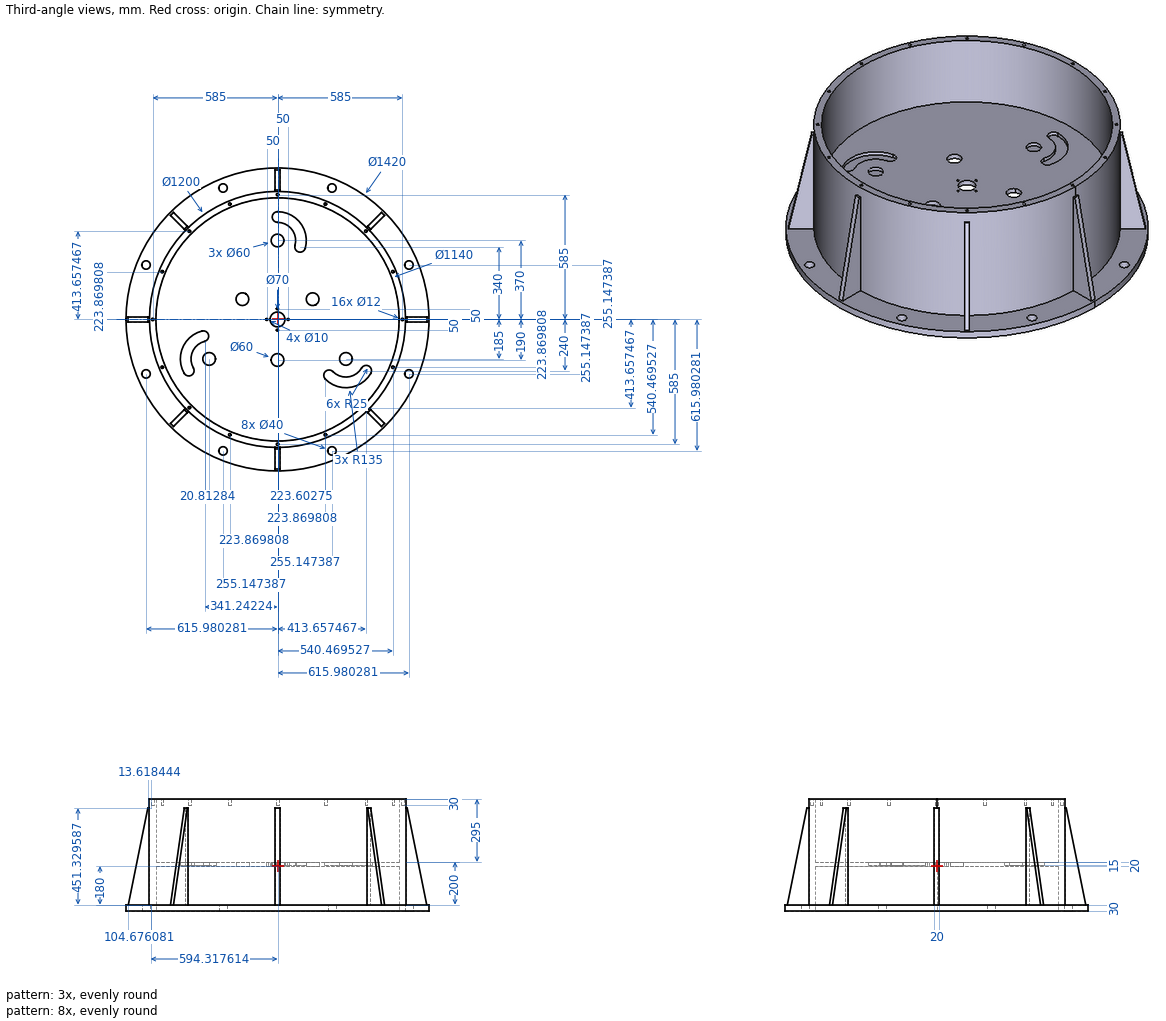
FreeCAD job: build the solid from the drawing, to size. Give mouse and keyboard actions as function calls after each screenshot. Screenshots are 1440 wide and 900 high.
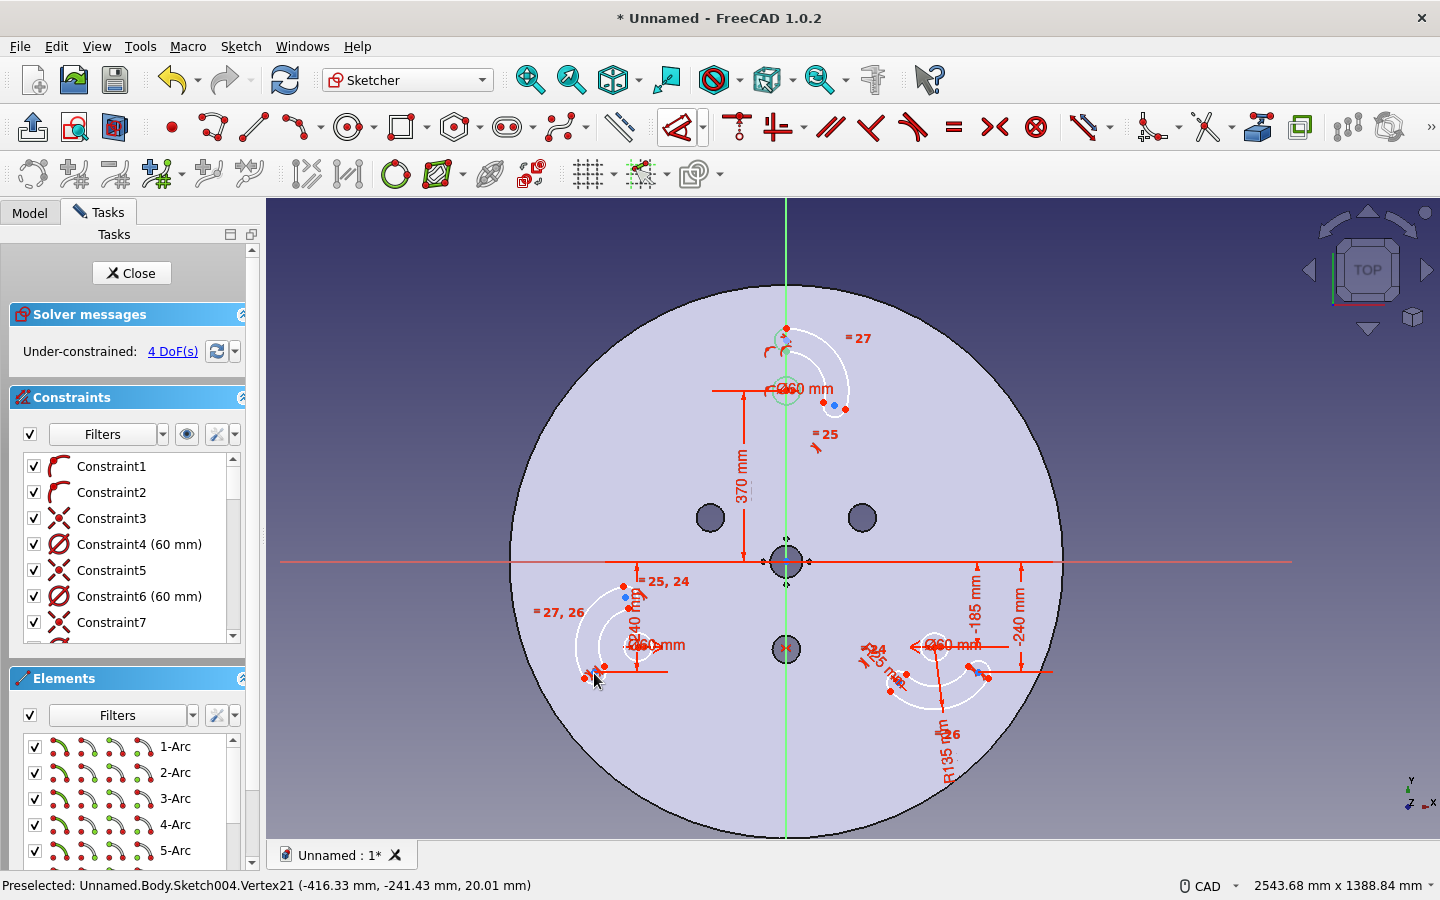
click(835, 406)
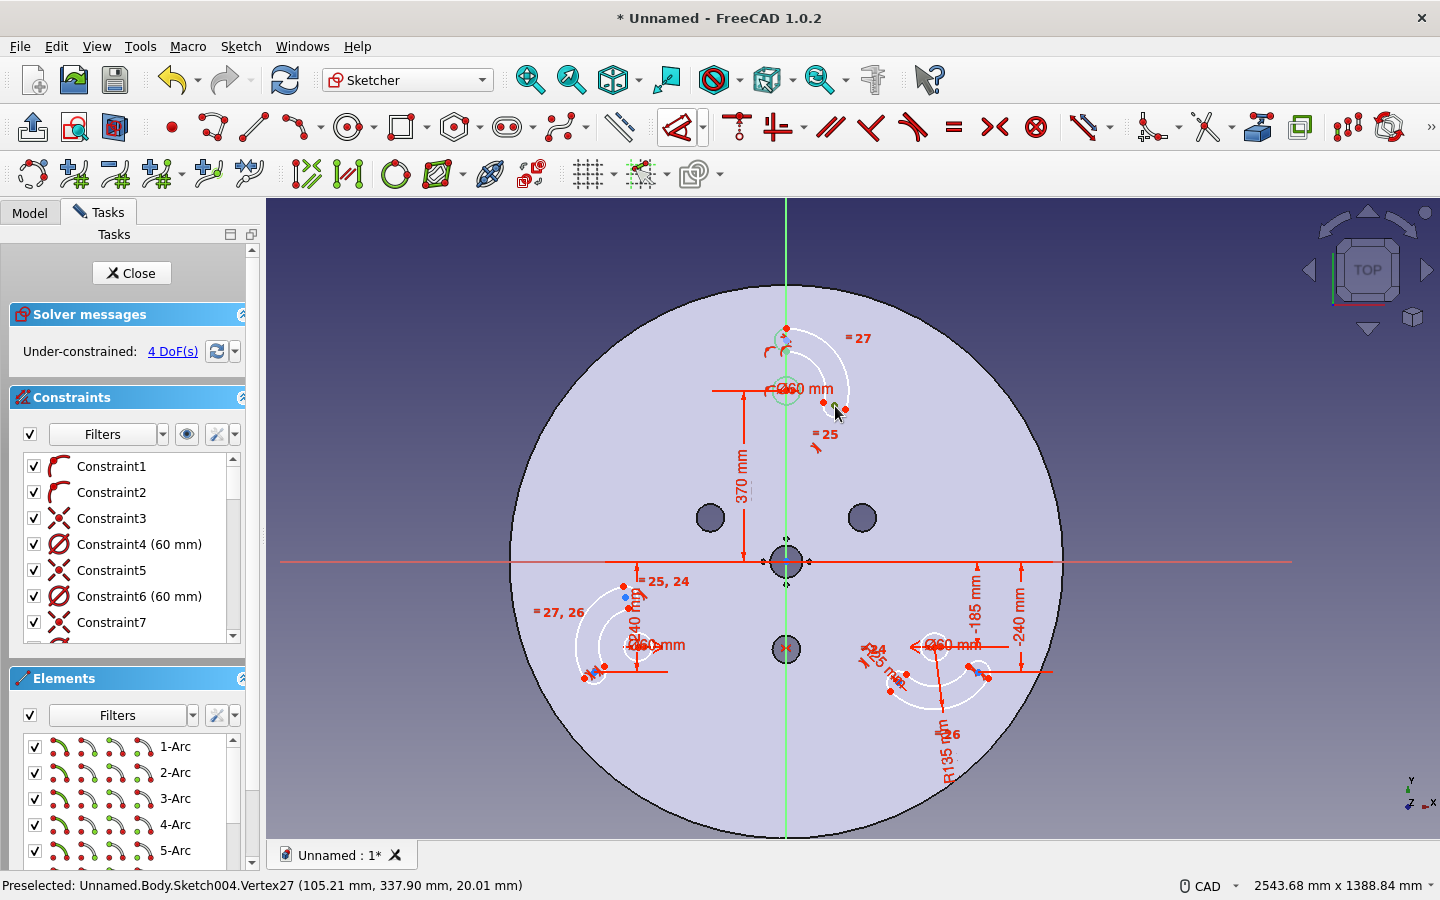
click(702, 128)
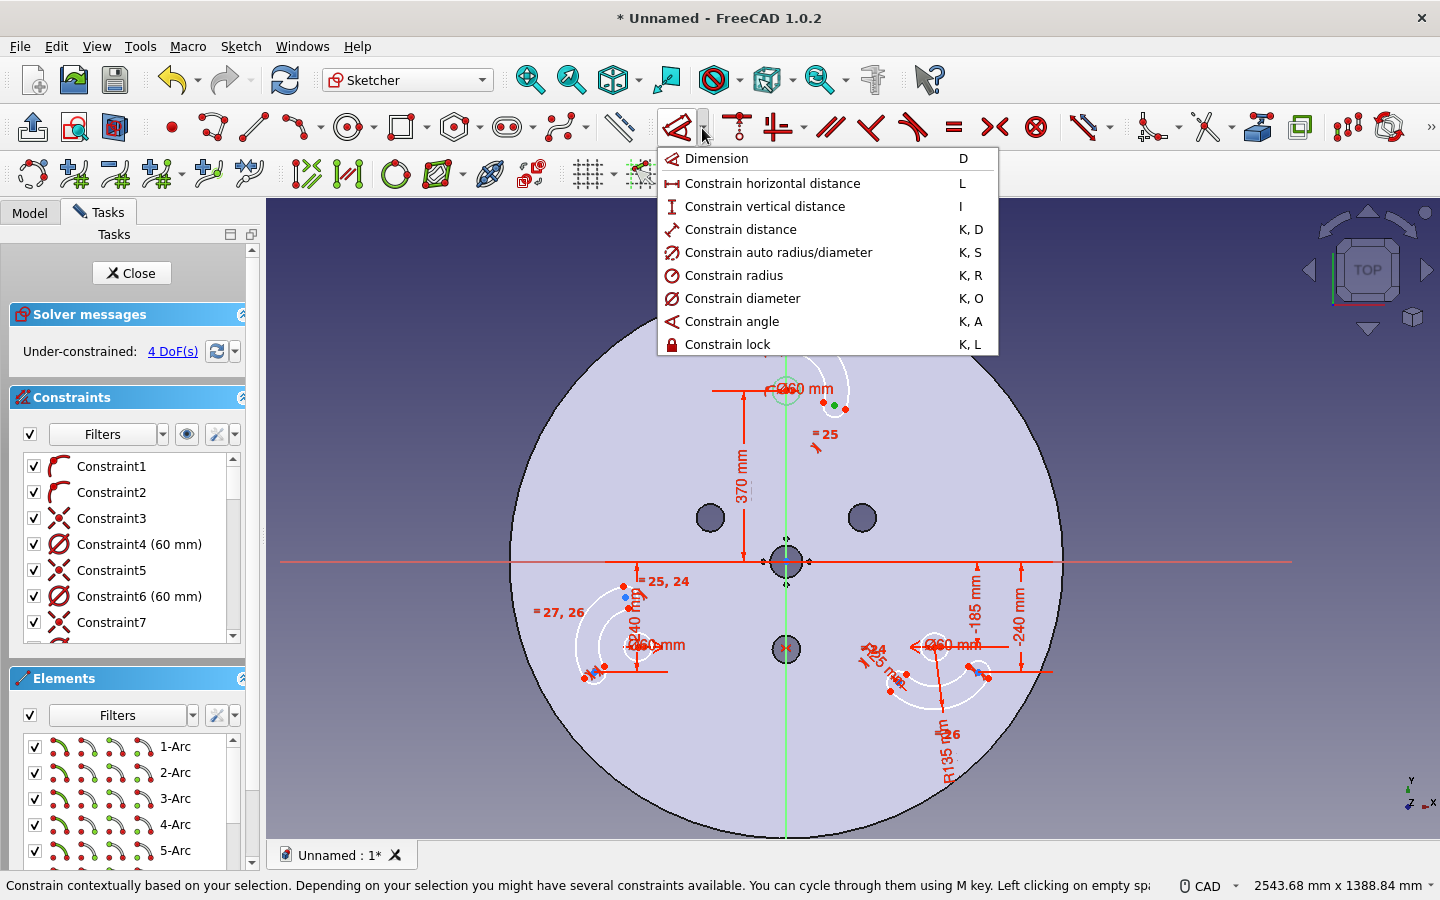
click(828, 206)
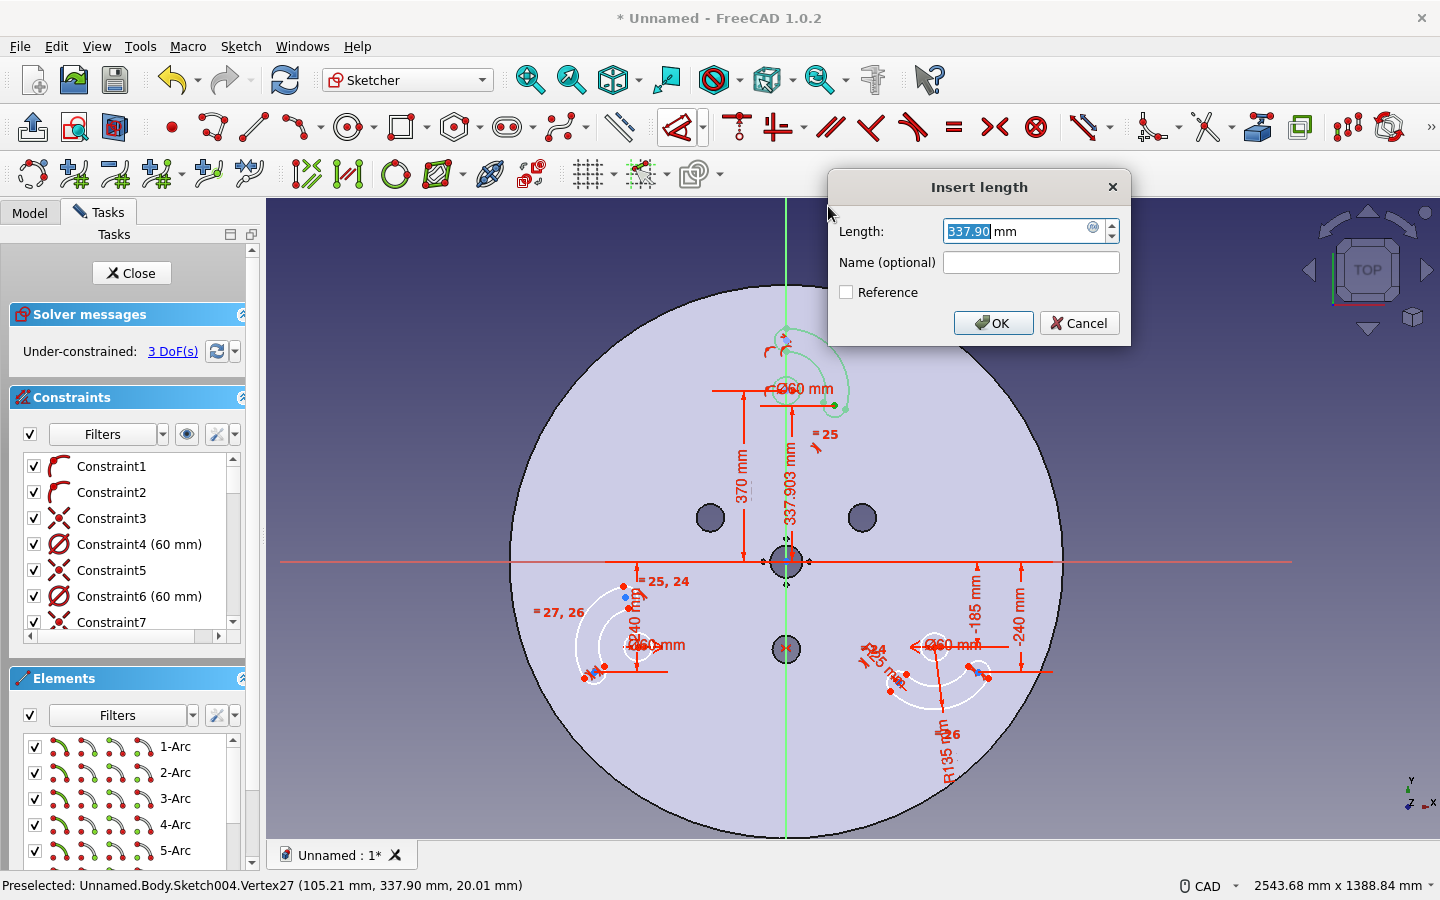
text(340)
key(Return)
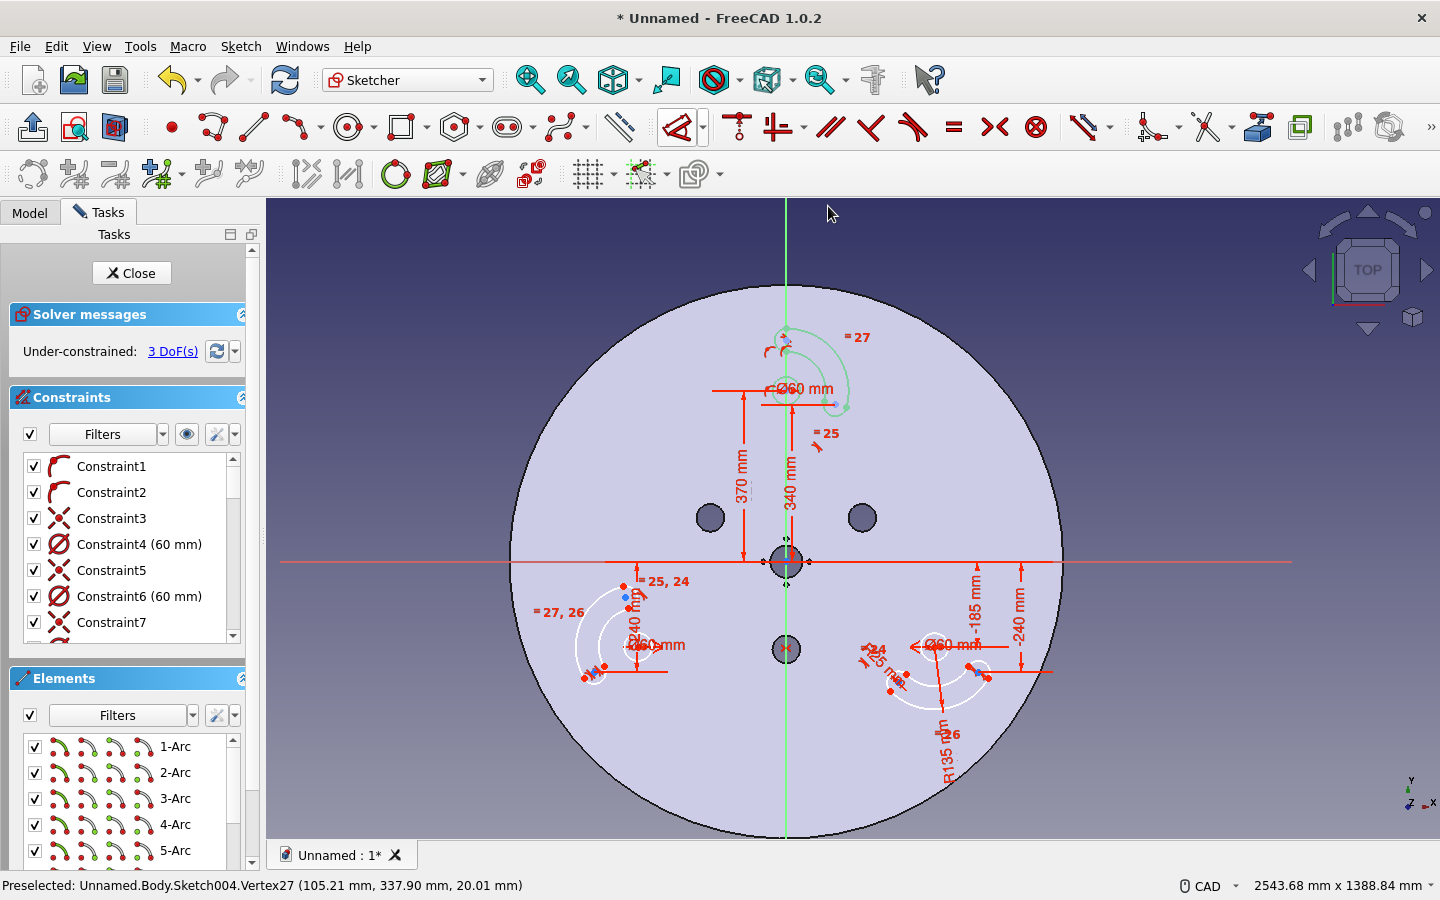
scroll(629, 609, up, 8)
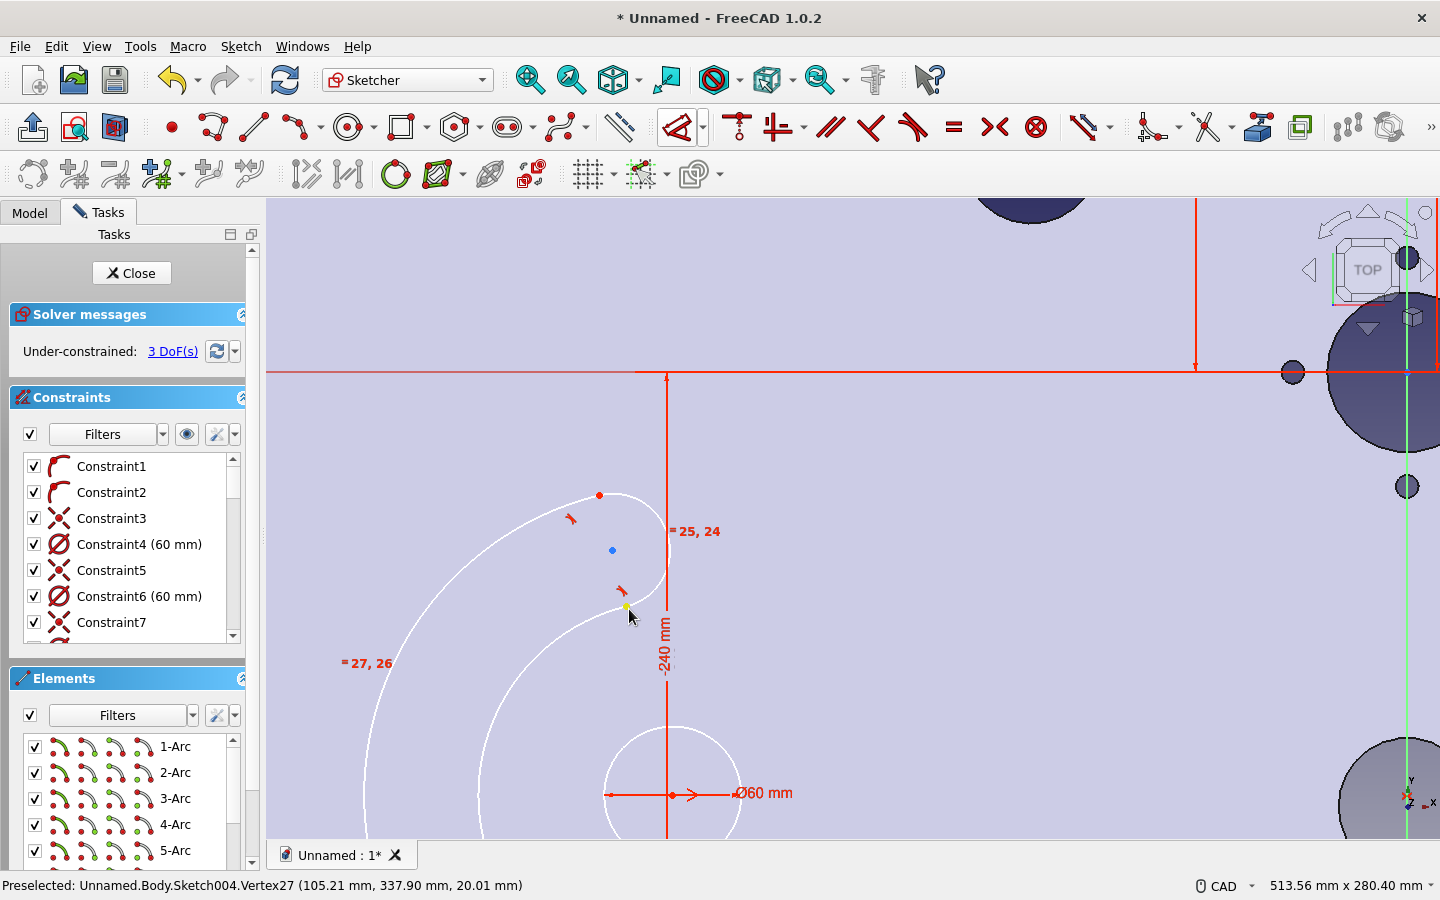
click(626, 606)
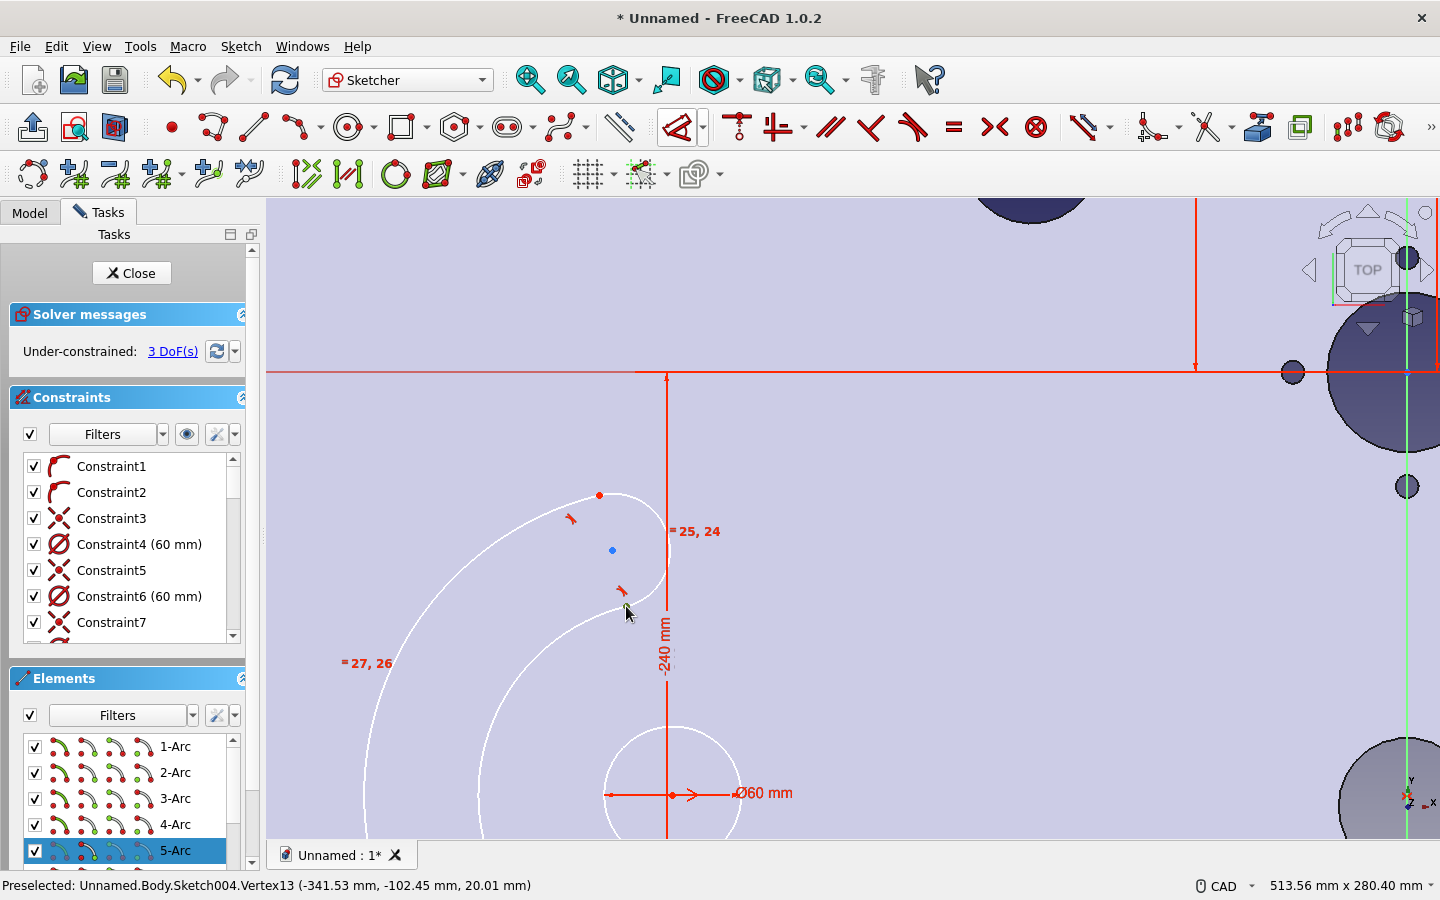
click(673, 795)